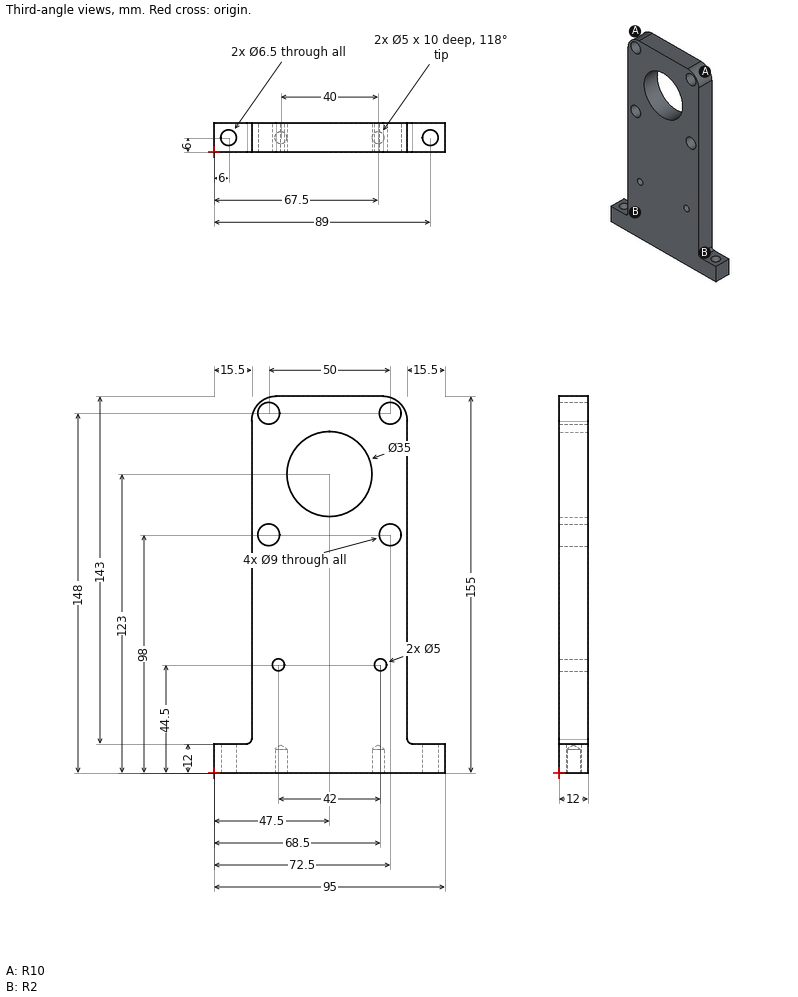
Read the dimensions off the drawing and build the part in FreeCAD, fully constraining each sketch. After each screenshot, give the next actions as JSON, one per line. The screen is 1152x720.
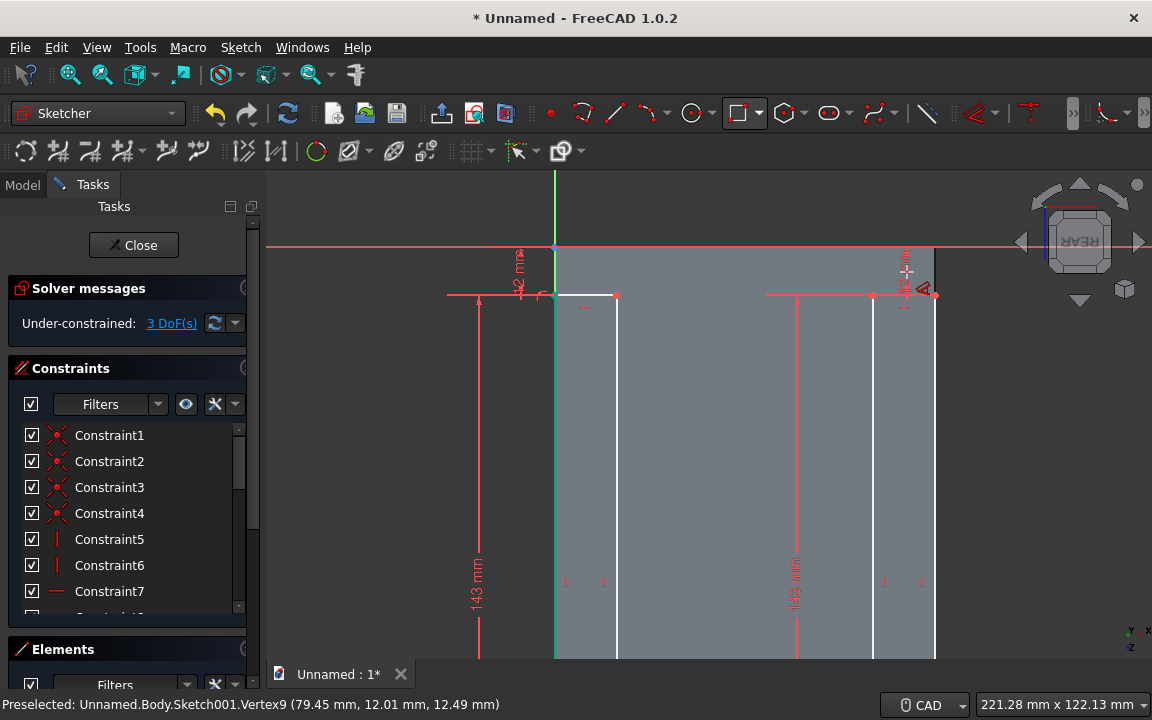
{"action": "scroll", "coordinate": [555, 298], "scroll_direction": "down", "scroll_amount": 4}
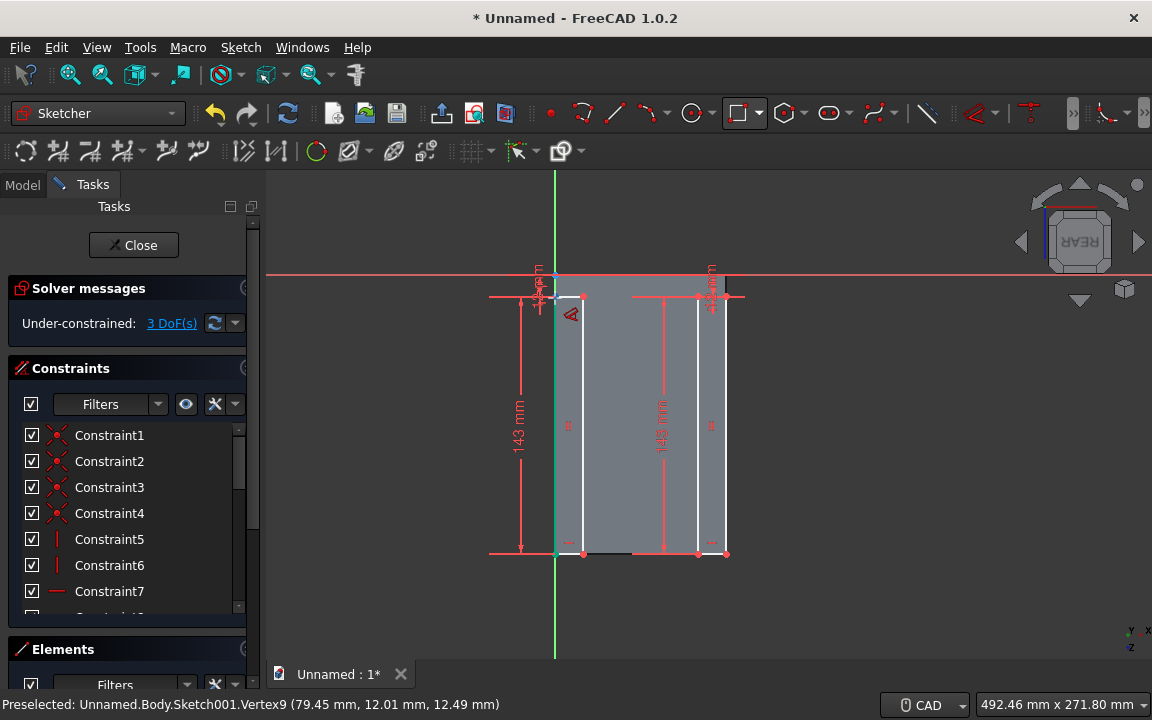
{"action": "left_click", "coordinate": [726, 554]}
{"action": "left_click", "coordinate": [641, 241]}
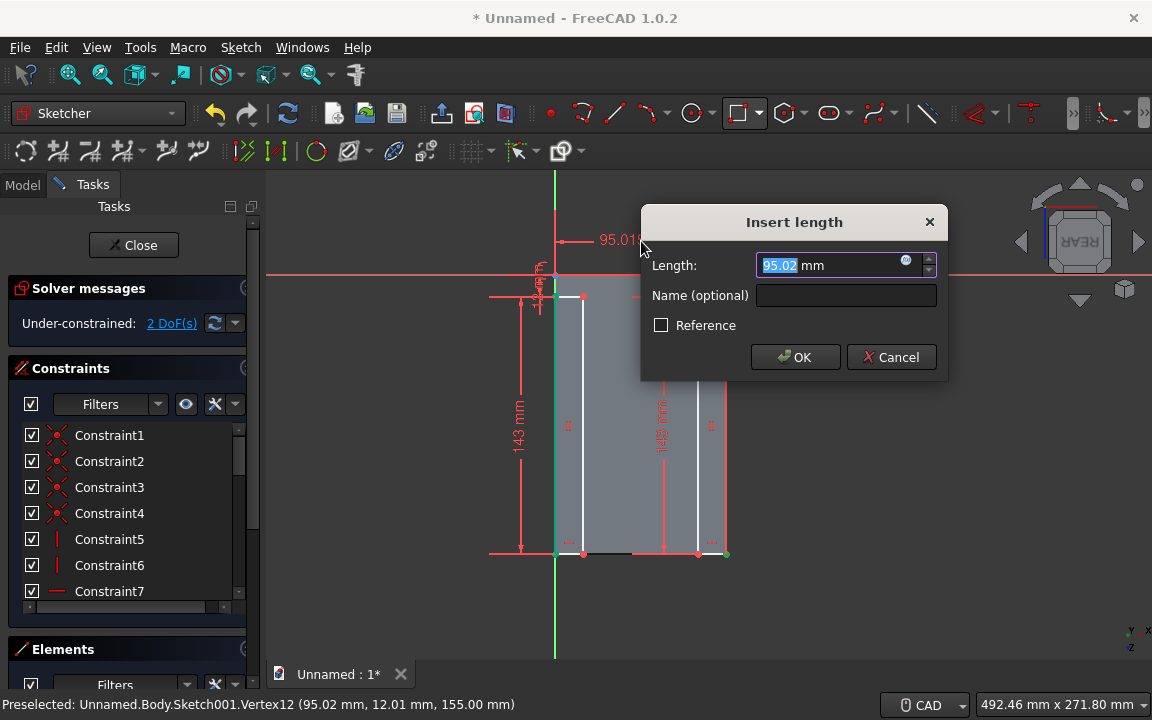
{"action": "type", "text": "95"}
{"action": "key", "text": "Return"}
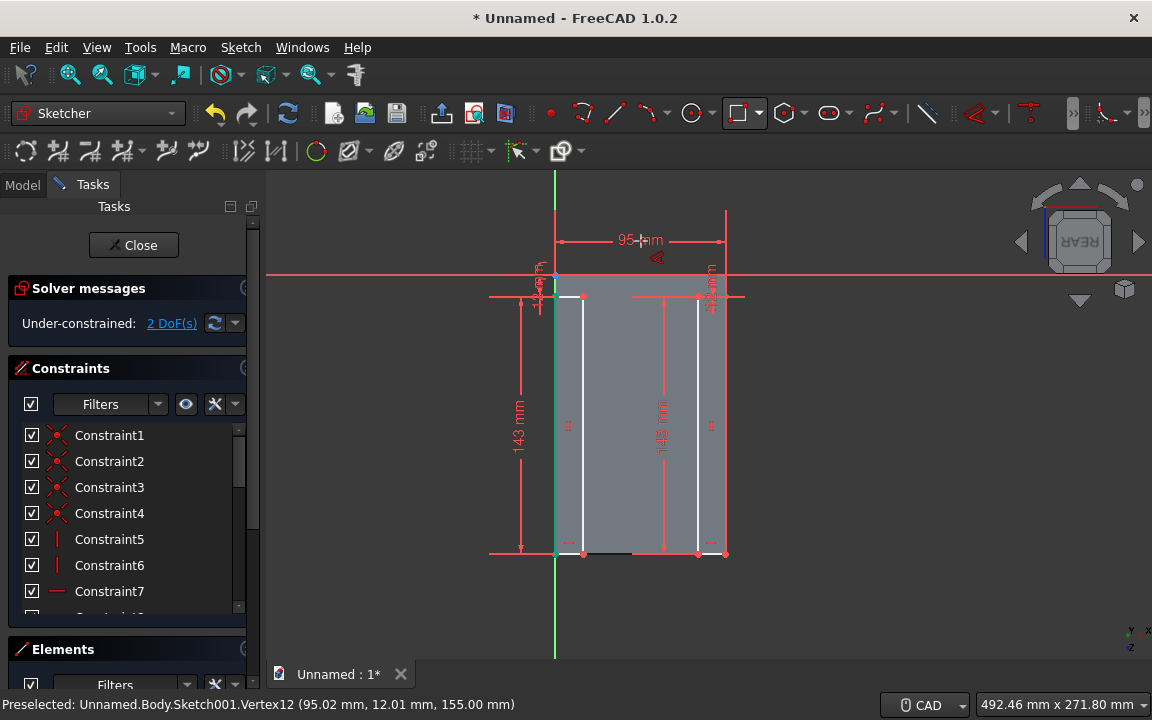
{"action": "scroll", "coordinate": [566, 554], "scroll_direction": "up", "scroll_amount": 2}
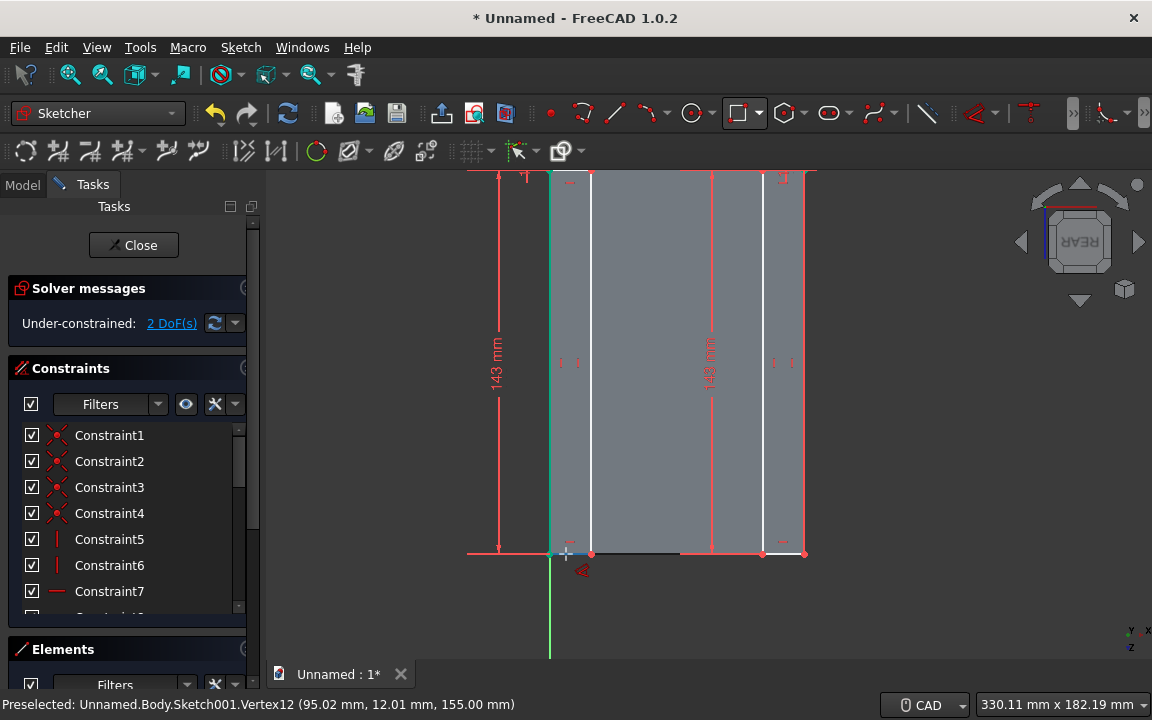
{"action": "left_click", "coordinate": [566, 554]}
{"action": "left_click", "coordinate": [570, 588]}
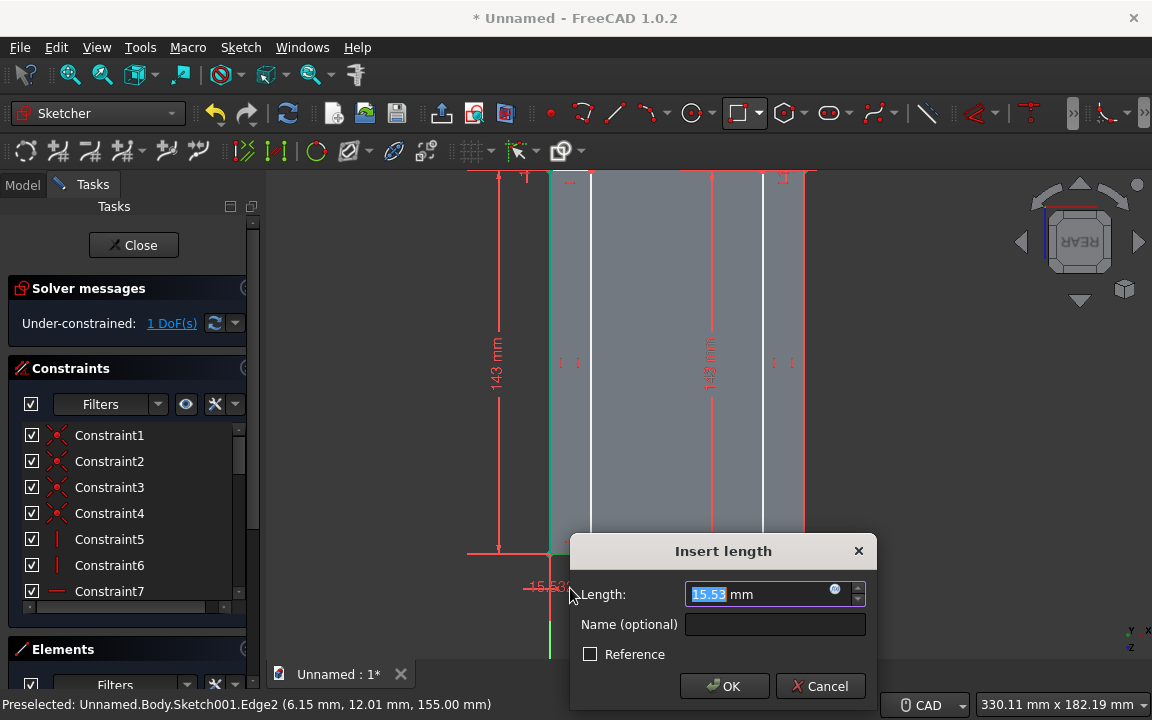
{"action": "type", "text": "15.5"}
{"action": "key", "text": "Return"}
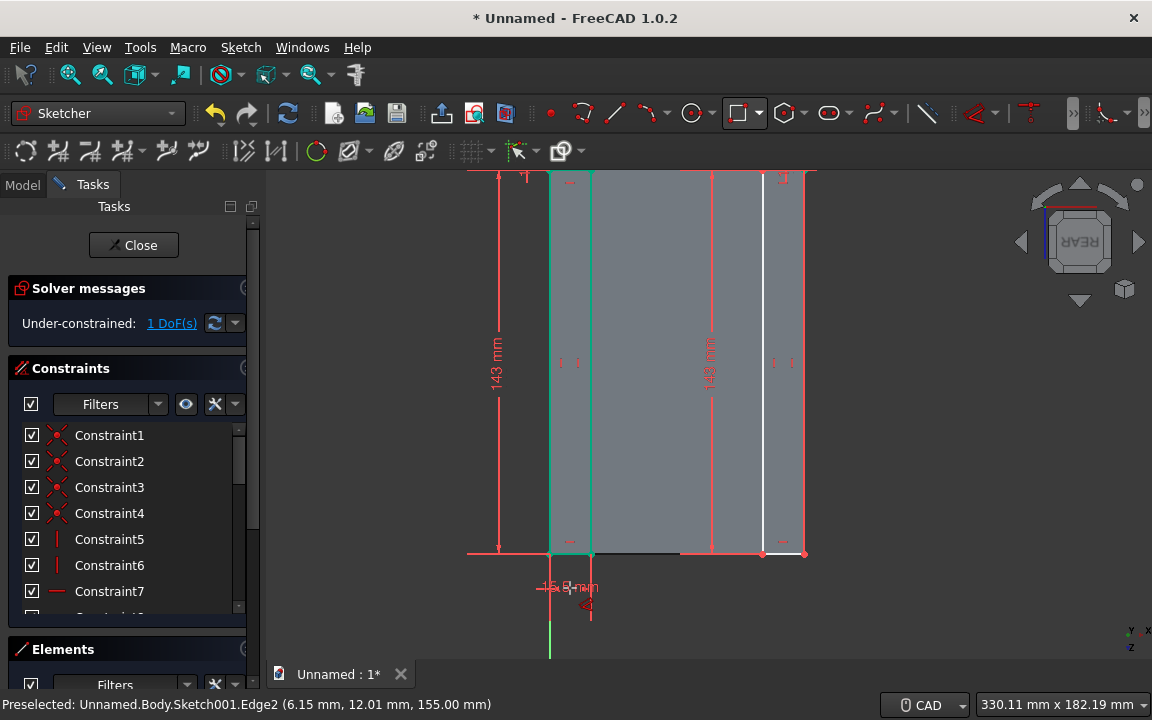
{"action": "left_click", "coordinate": [775, 554]}
{"action": "left_click", "coordinate": [784, 588]}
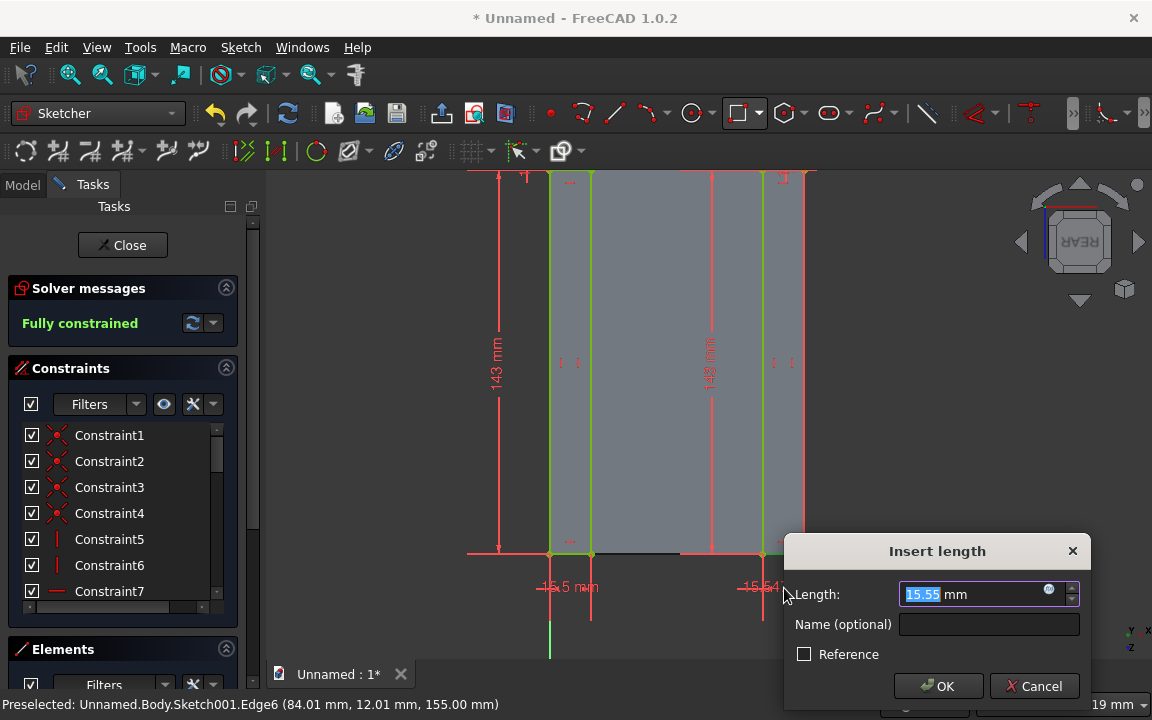
{"action": "type", "text": "15.5"}
{"action": "key", "text": "Return"}
{"action": "key", "text": "Escape"}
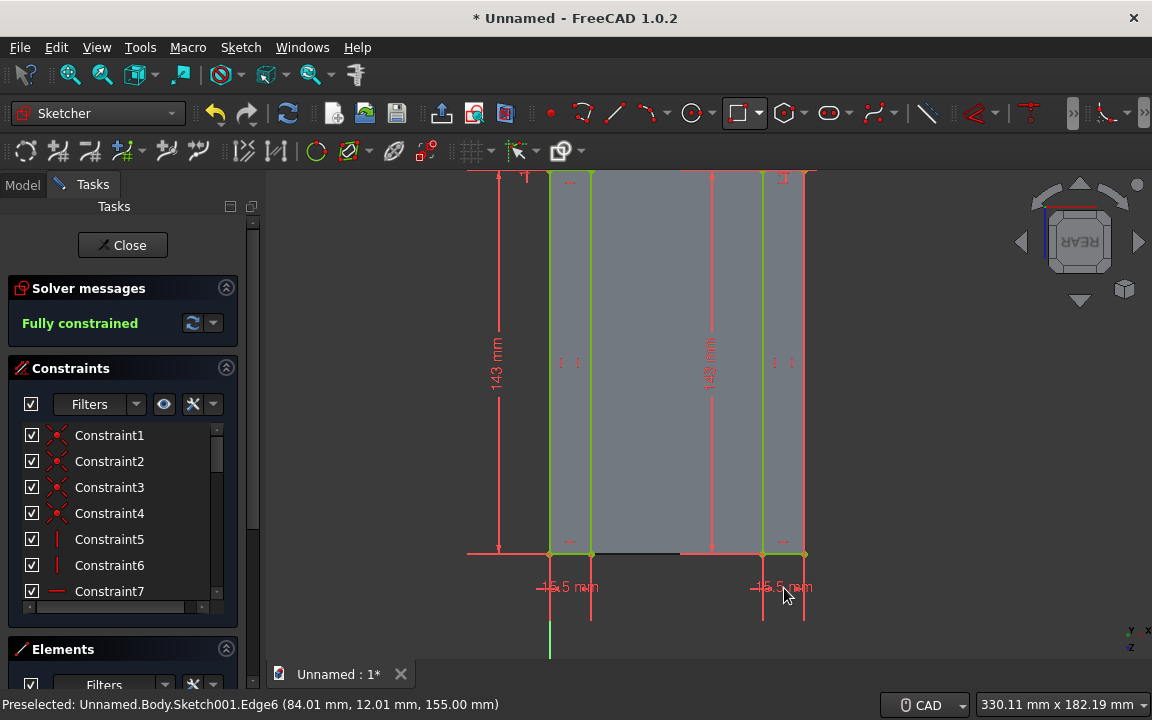
{"action": "left_click", "coordinate": [123, 245]}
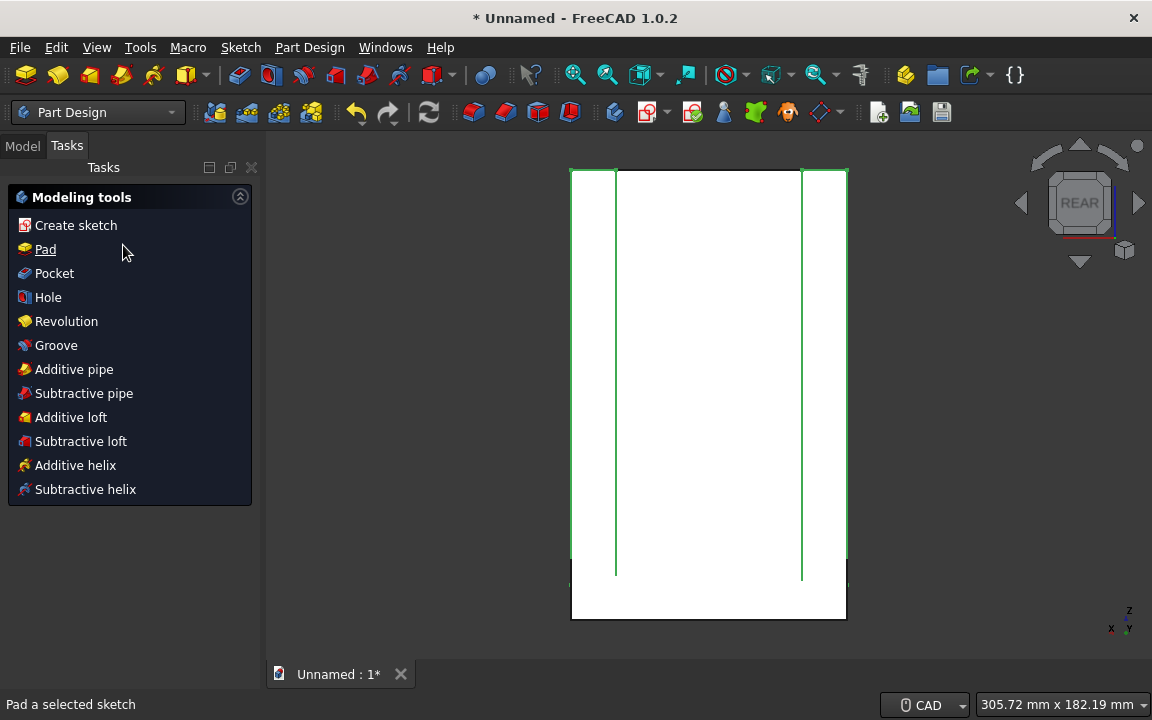
{"action": "left_click", "coordinate": [240, 76]}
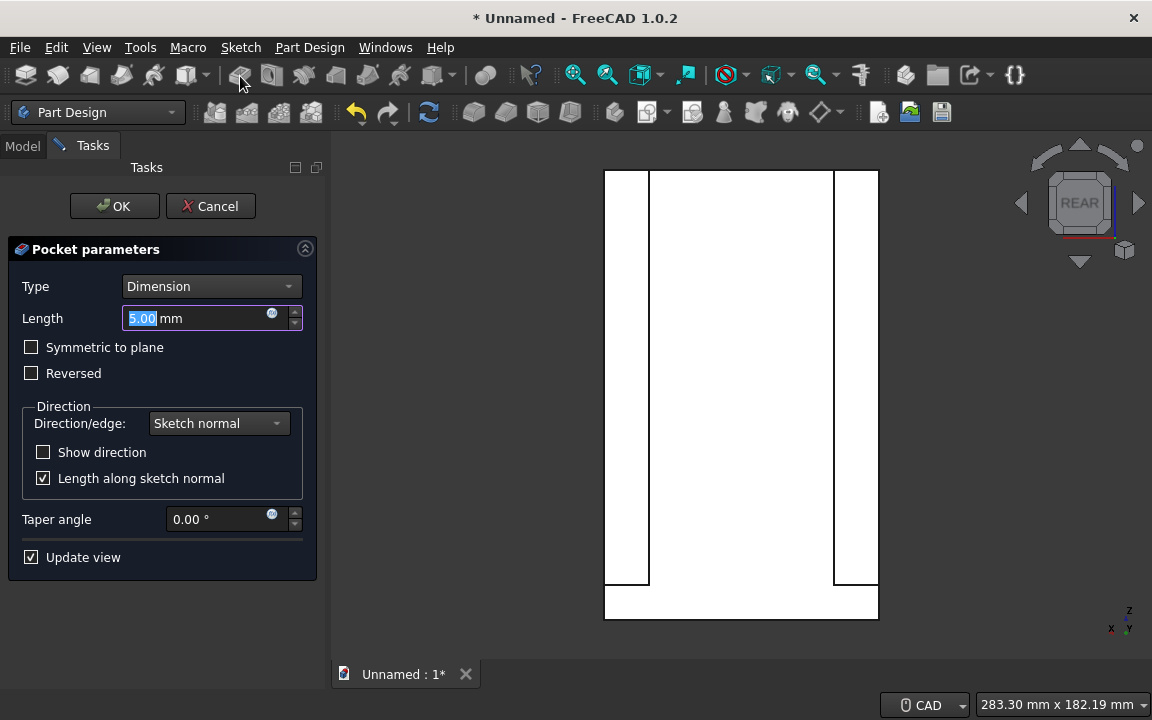
{"action": "left_click", "coordinate": [212, 286]}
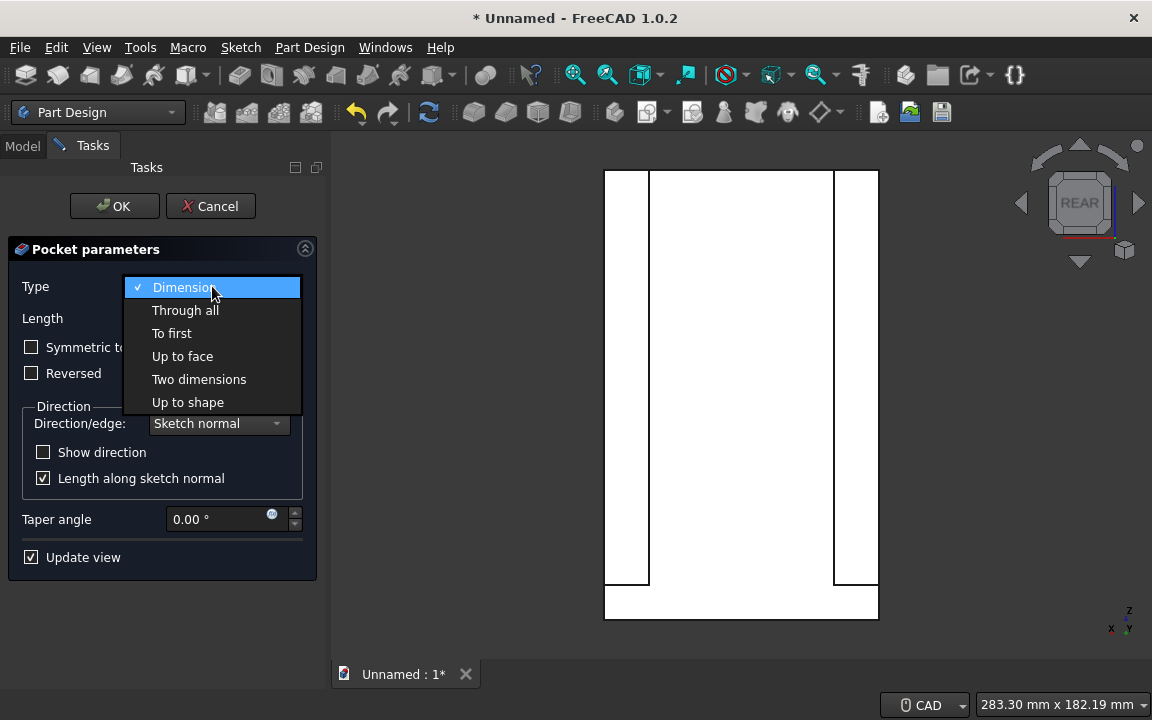
{"action": "left_click", "coordinate": [212, 310]}